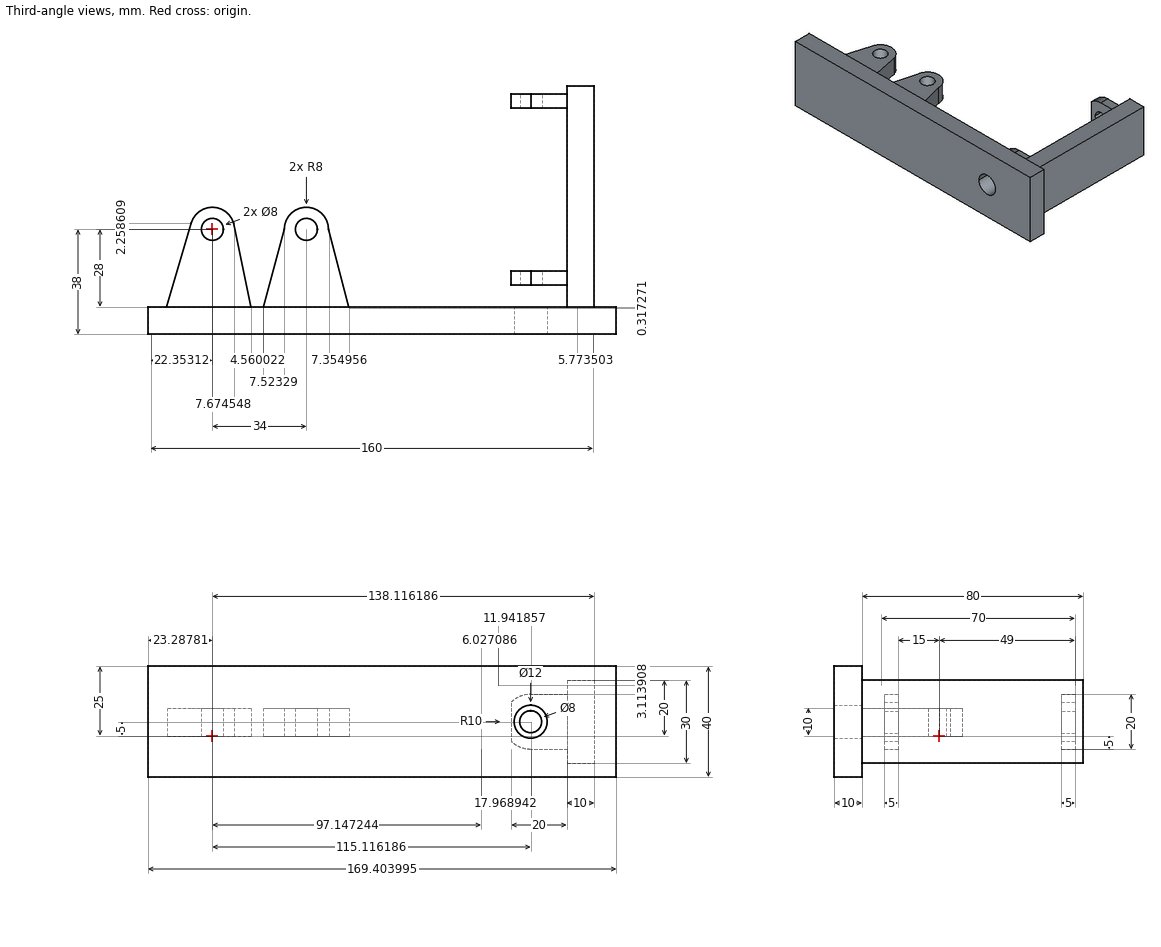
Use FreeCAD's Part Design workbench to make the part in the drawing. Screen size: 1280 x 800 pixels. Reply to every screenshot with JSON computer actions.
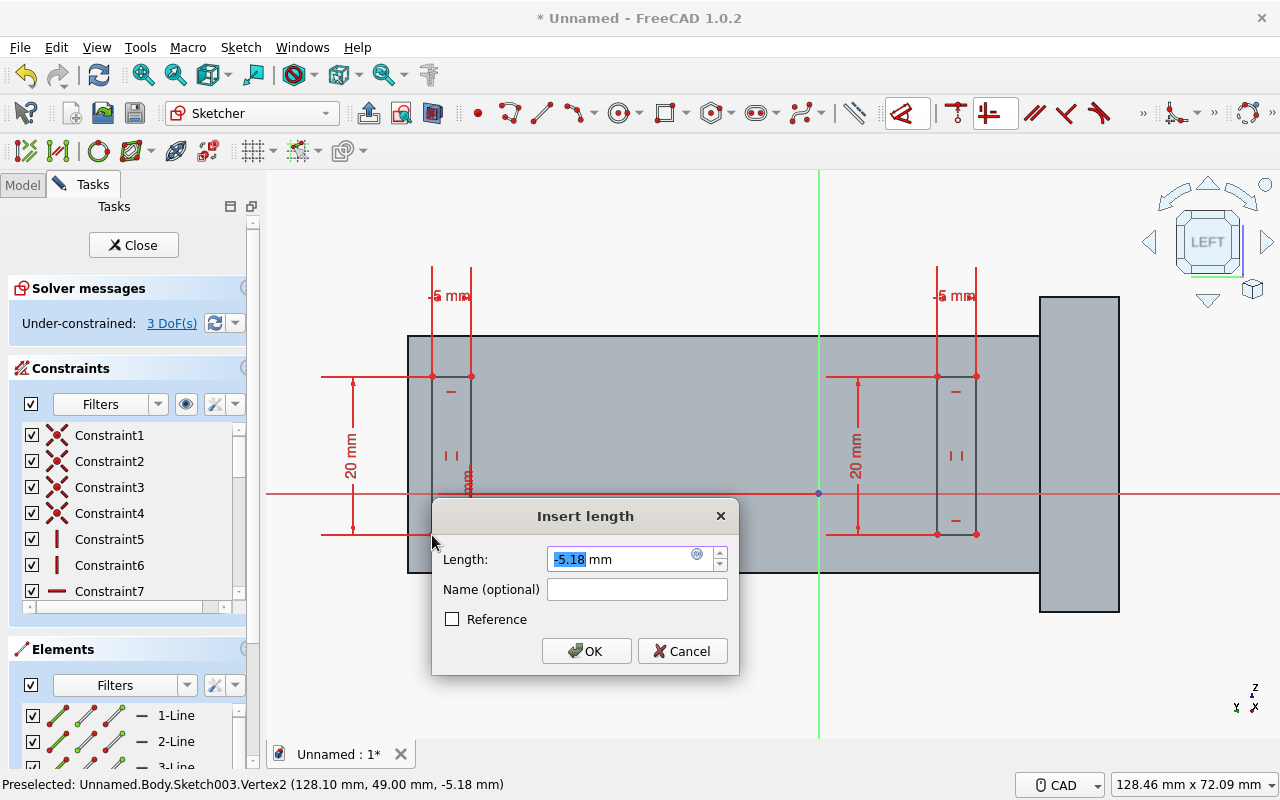
{"action": "type", "text": "-5"}
{"action": "key", "text": "Return"}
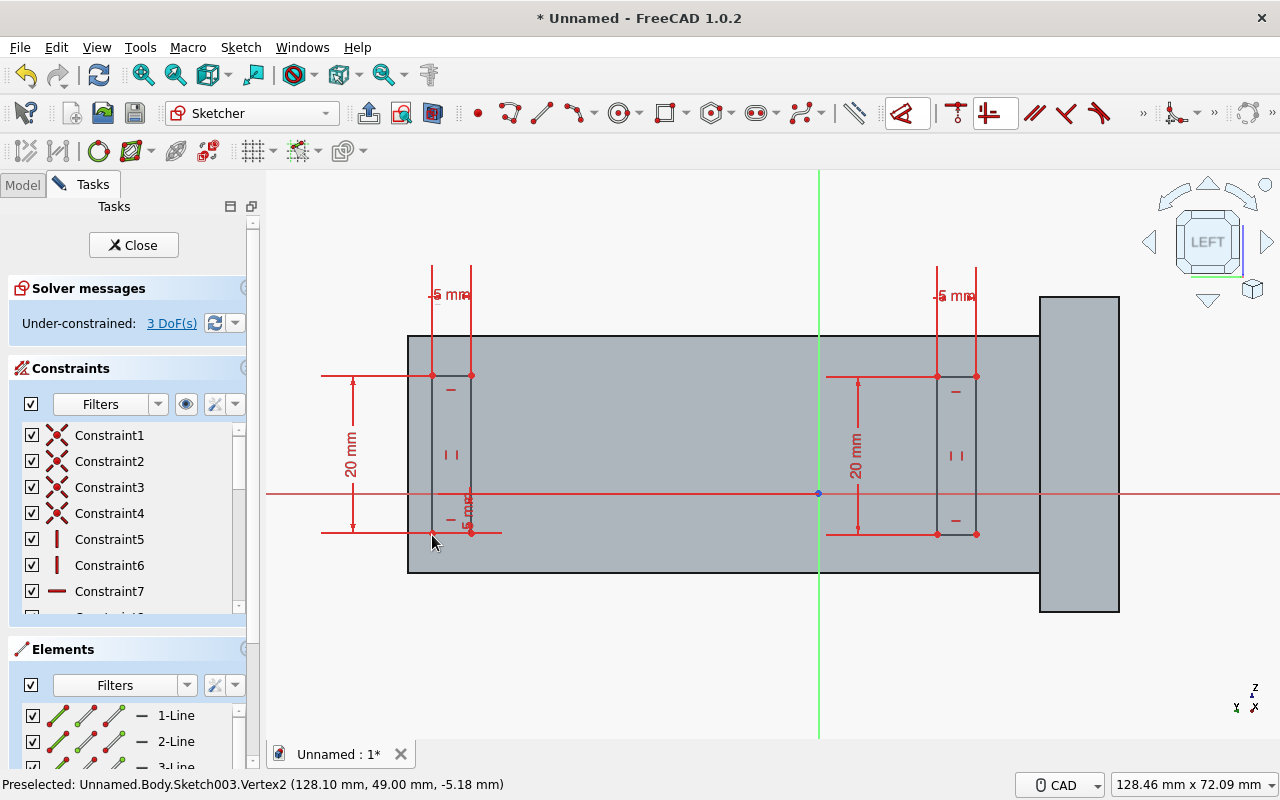
{"action": "left_click", "coordinate": [937, 535]}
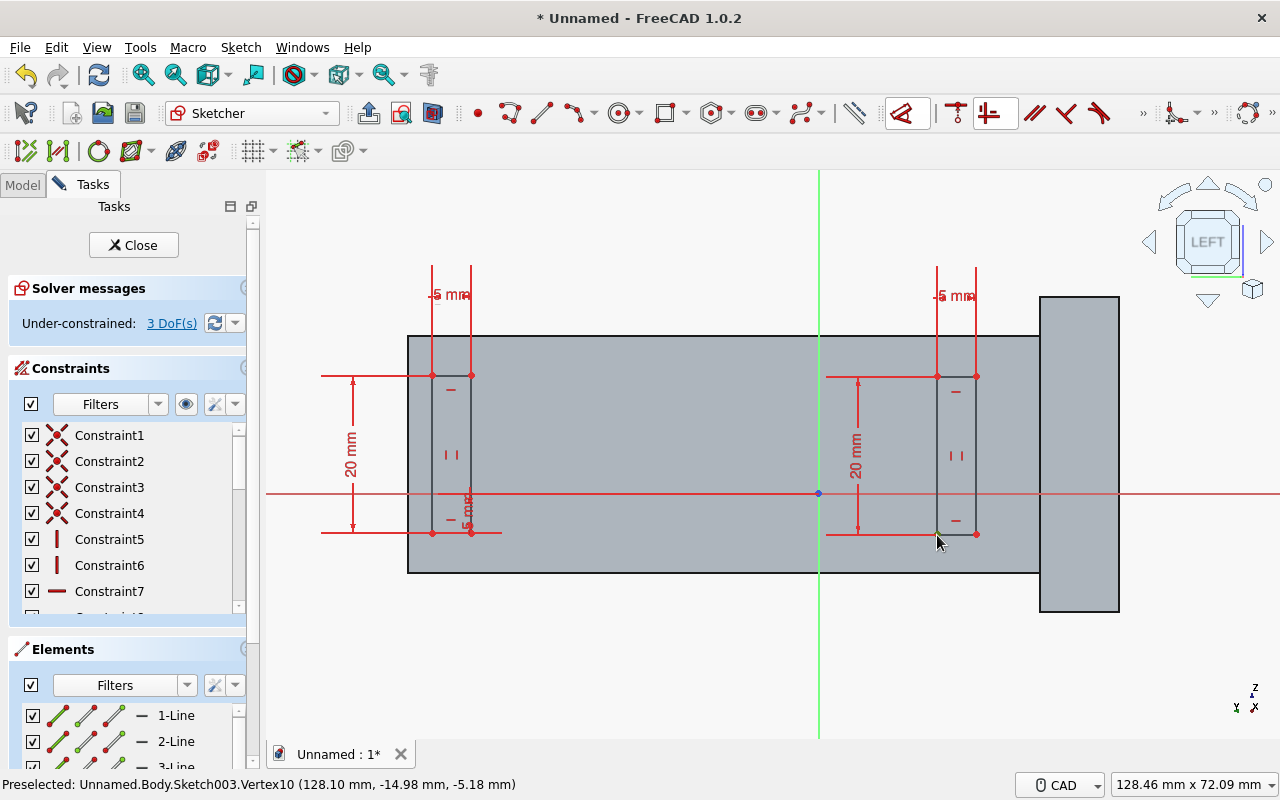
{"action": "left_click", "coordinate": [924, 114]}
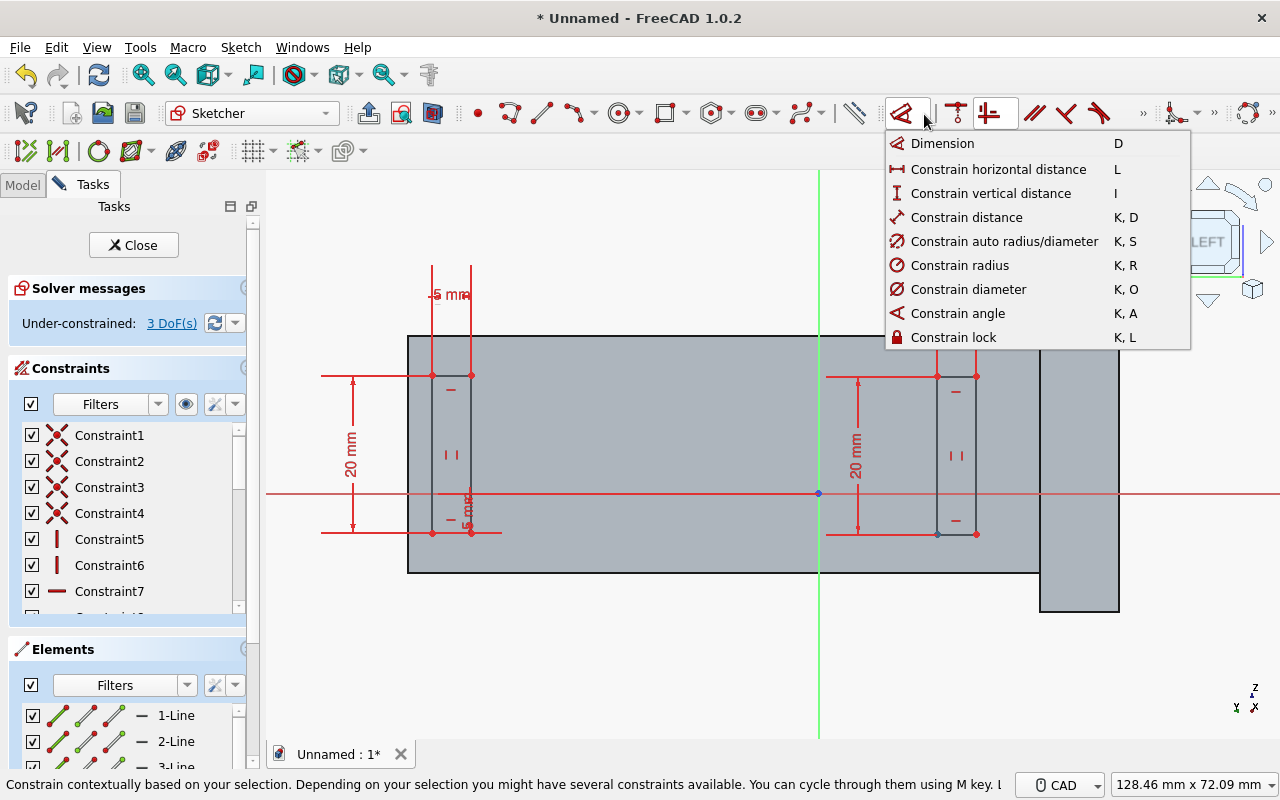
{"action": "left_click", "coordinate": [1038, 193]}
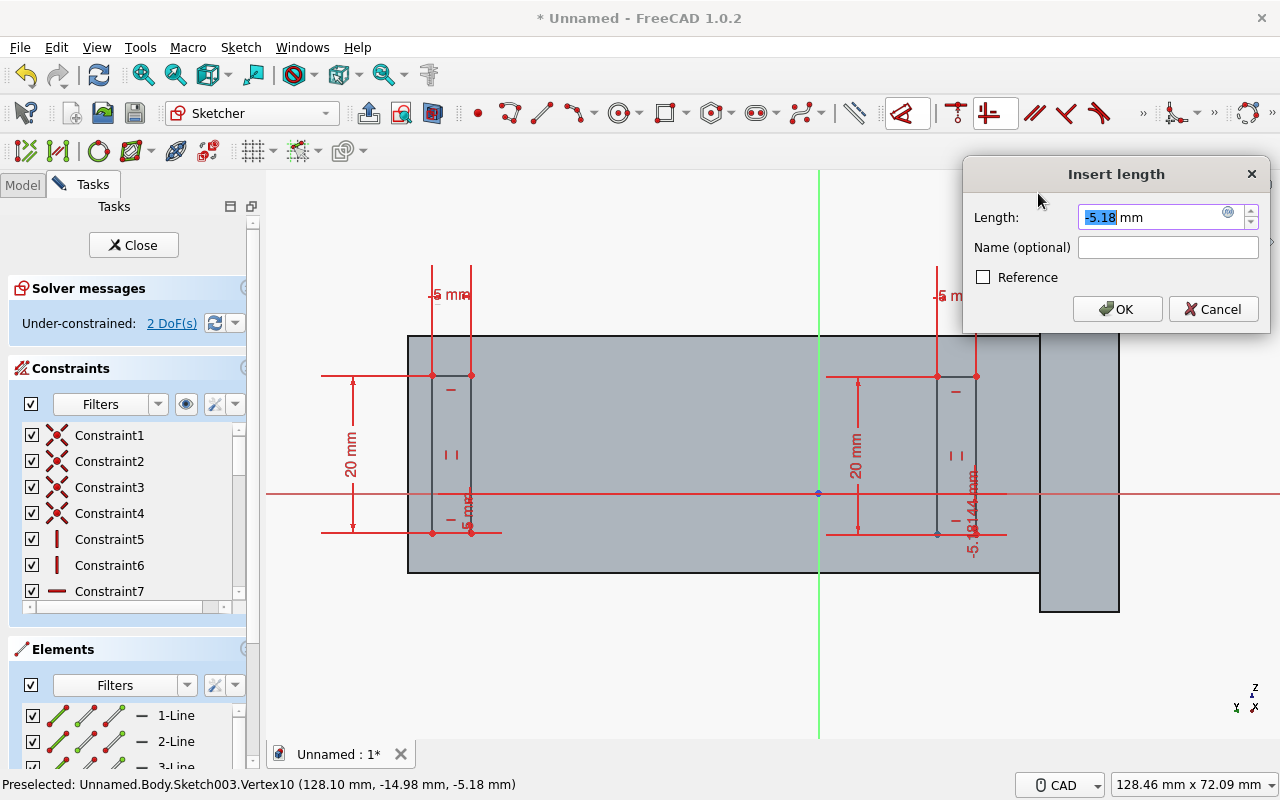
{"action": "type", "text": "-5"}
{"action": "key", "text": "Return"}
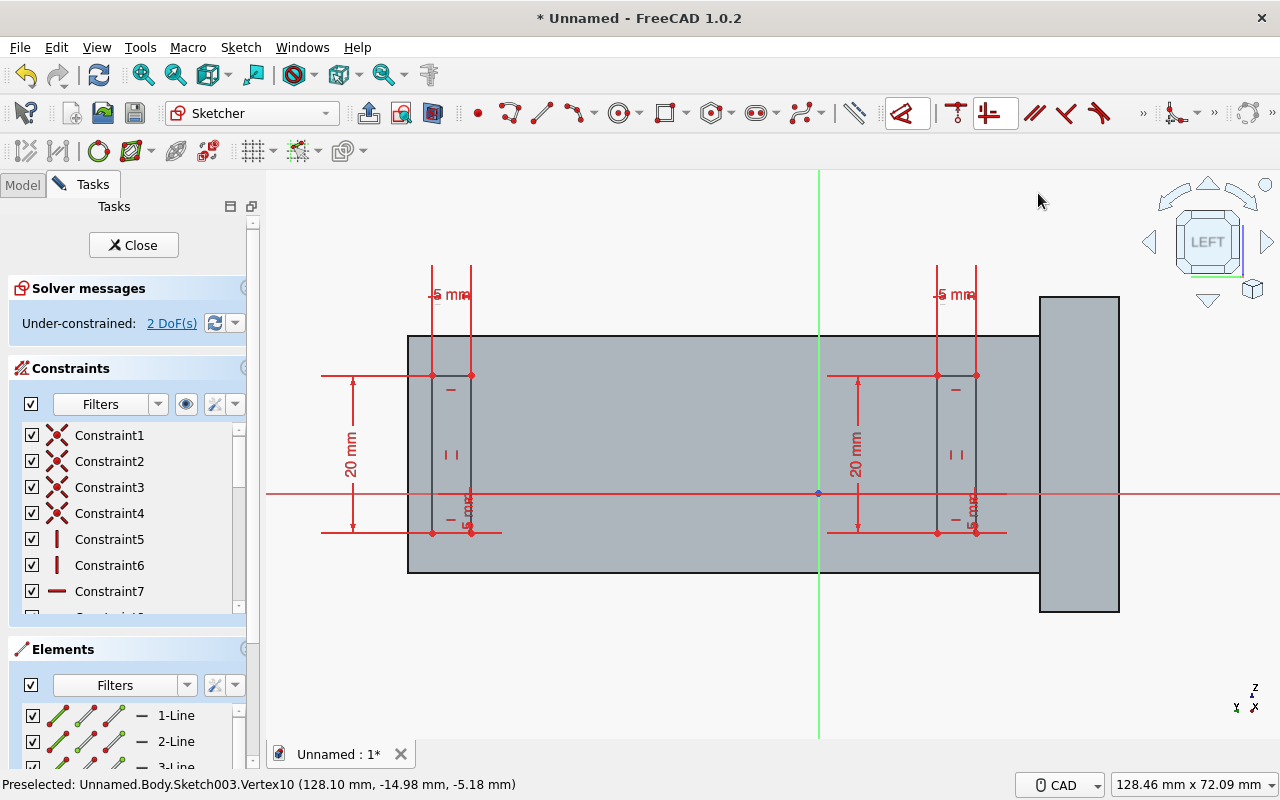
{"action": "left_click", "coordinate": [432, 376]}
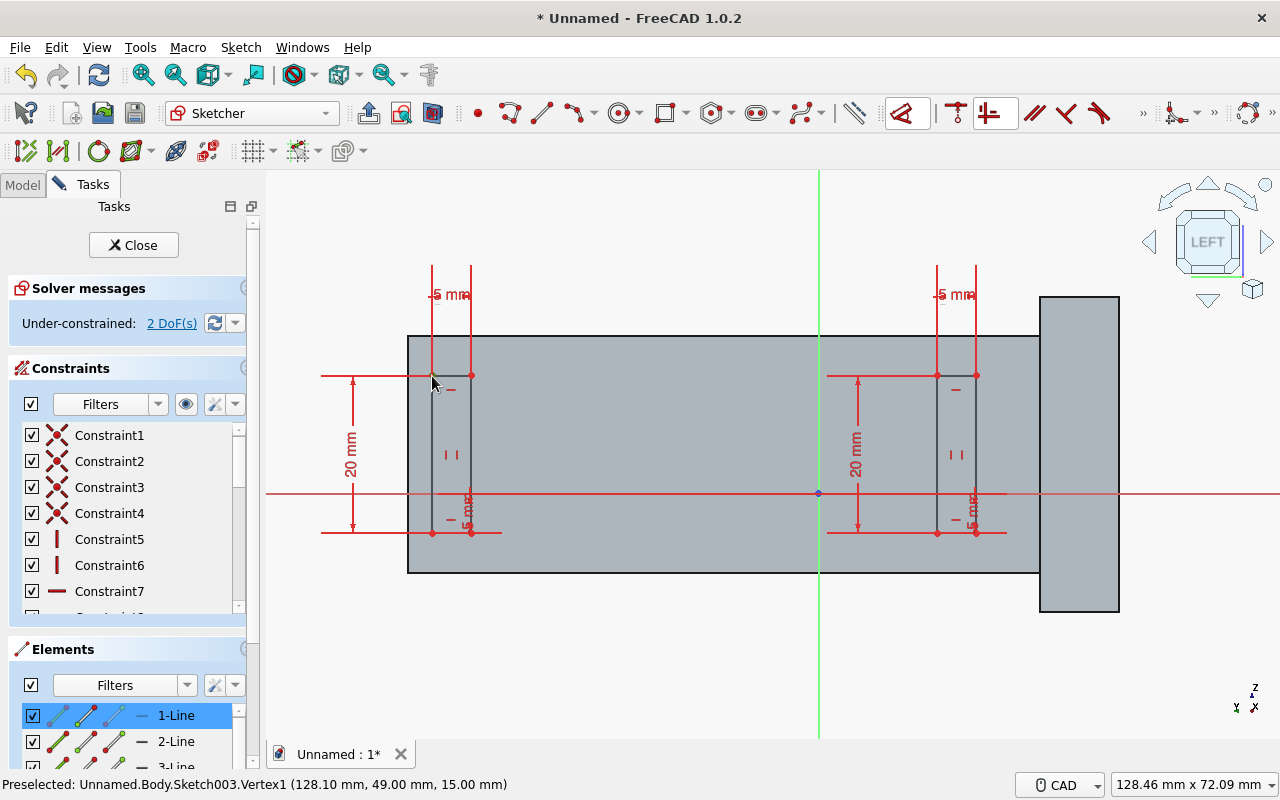
{"action": "left_click", "coordinate": [924, 114]}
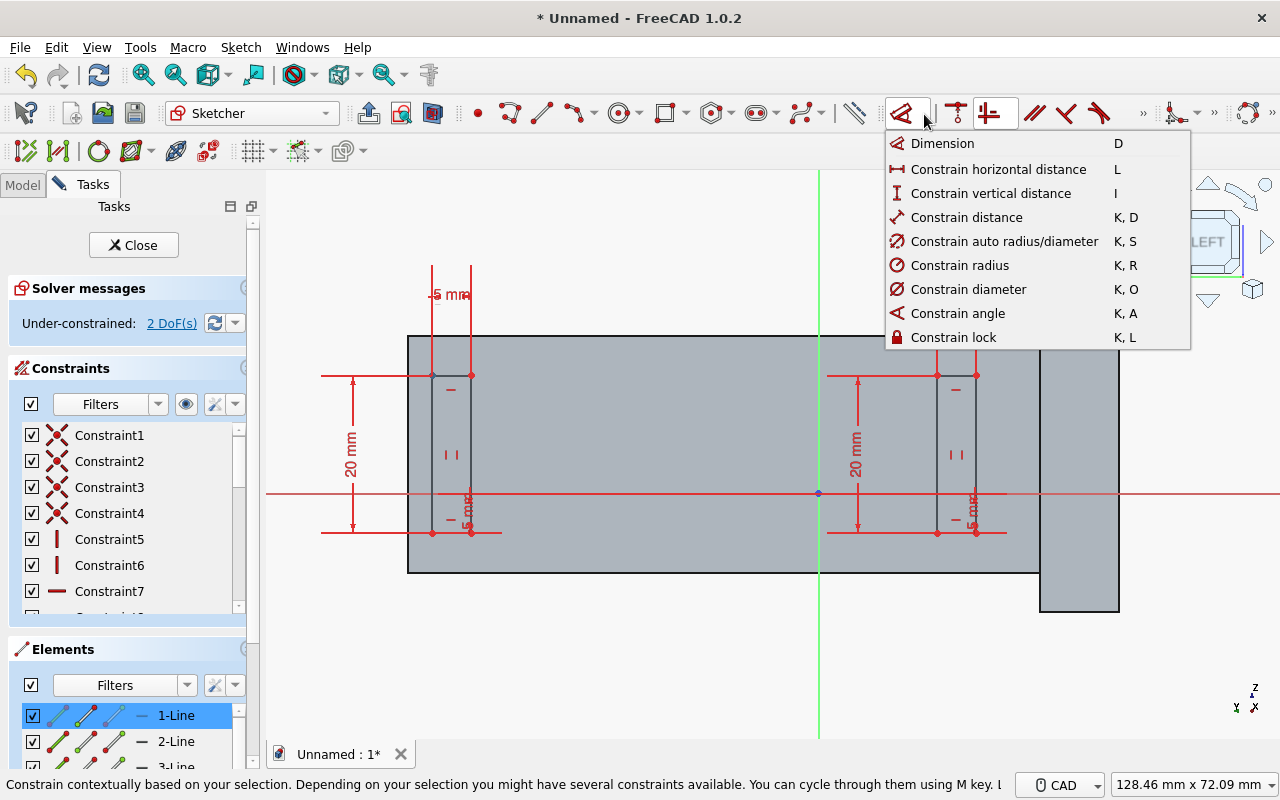
{"action": "left_click", "coordinate": [1038, 169]}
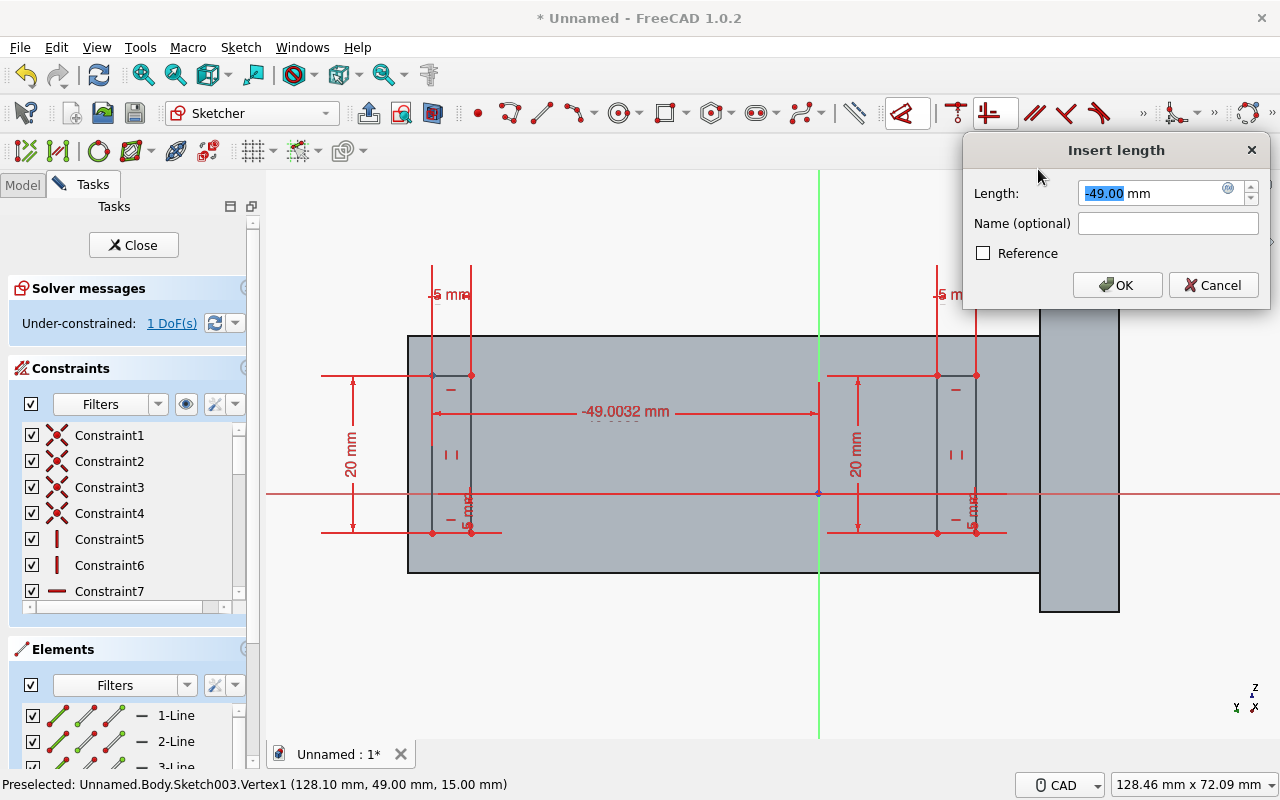
{"action": "type", "text": "-49"}
{"action": "key", "text": "Return"}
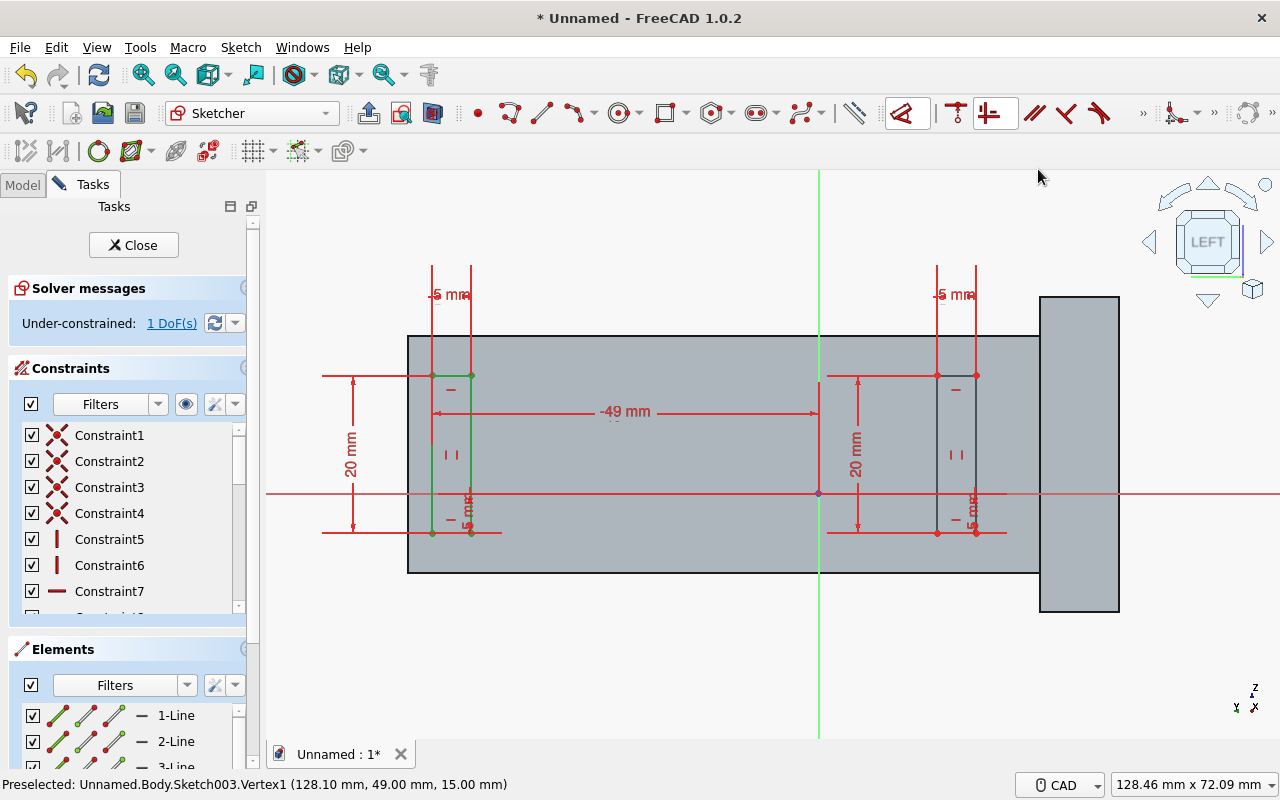
{"action": "left_click", "coordinate": [937, 376]}